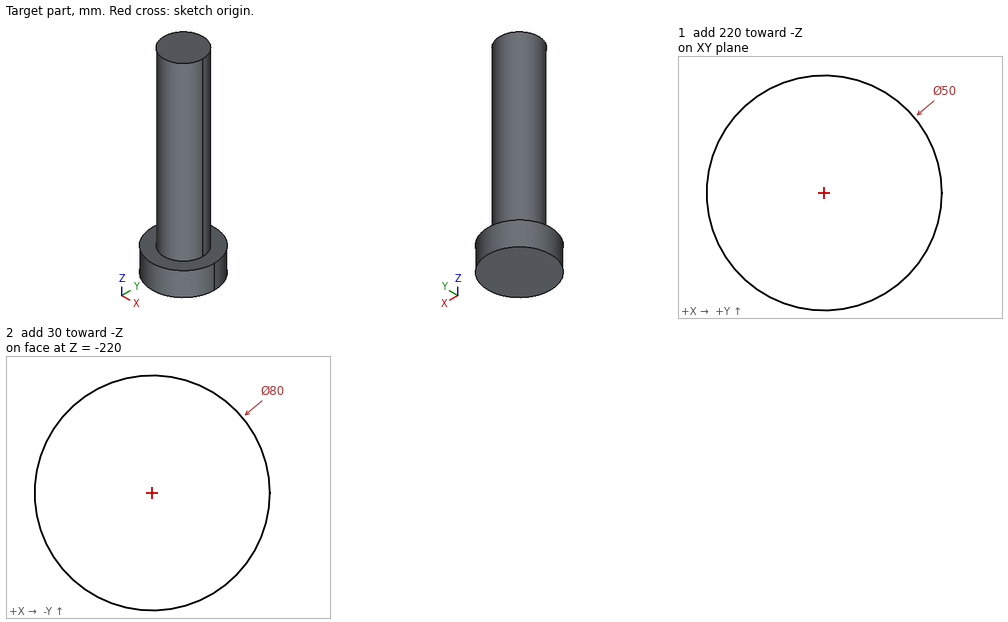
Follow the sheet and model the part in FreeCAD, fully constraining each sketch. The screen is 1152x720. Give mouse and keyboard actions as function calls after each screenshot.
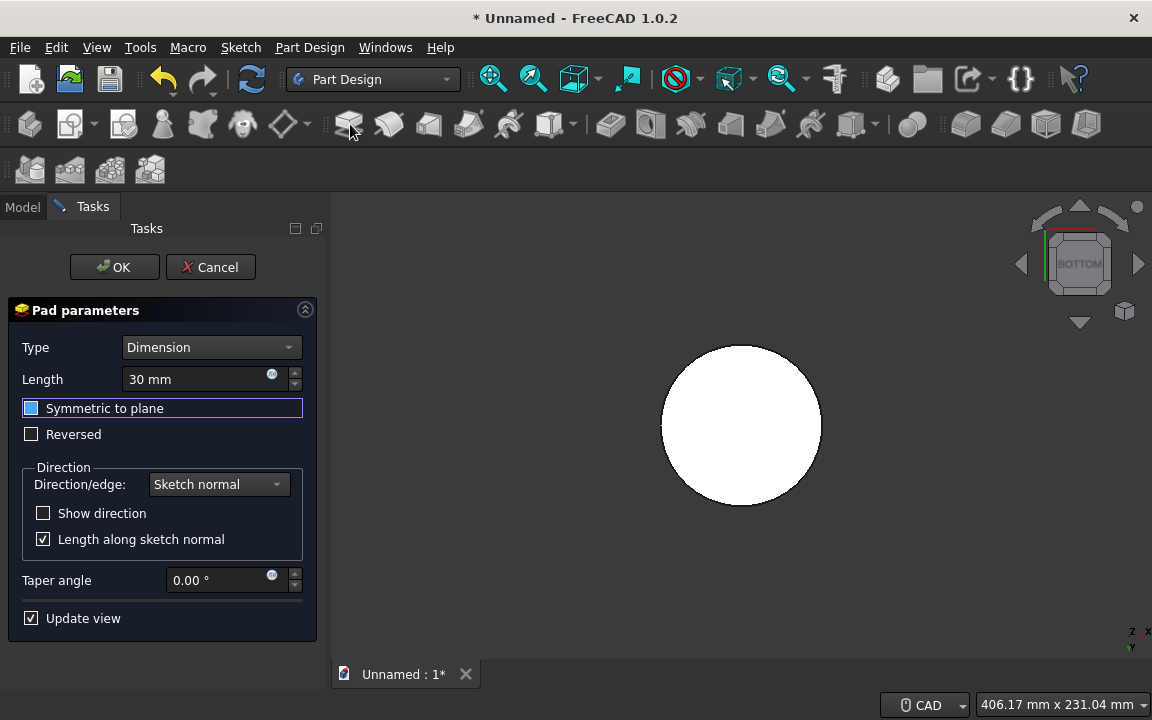
click(115, 267)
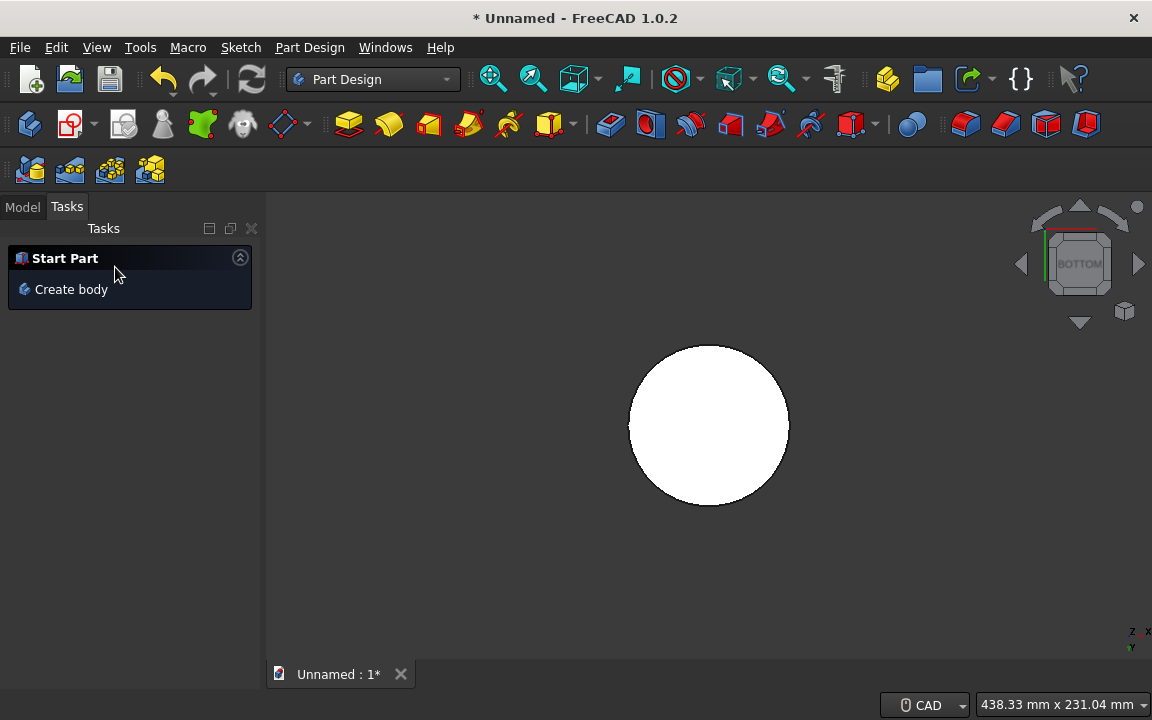
key(0)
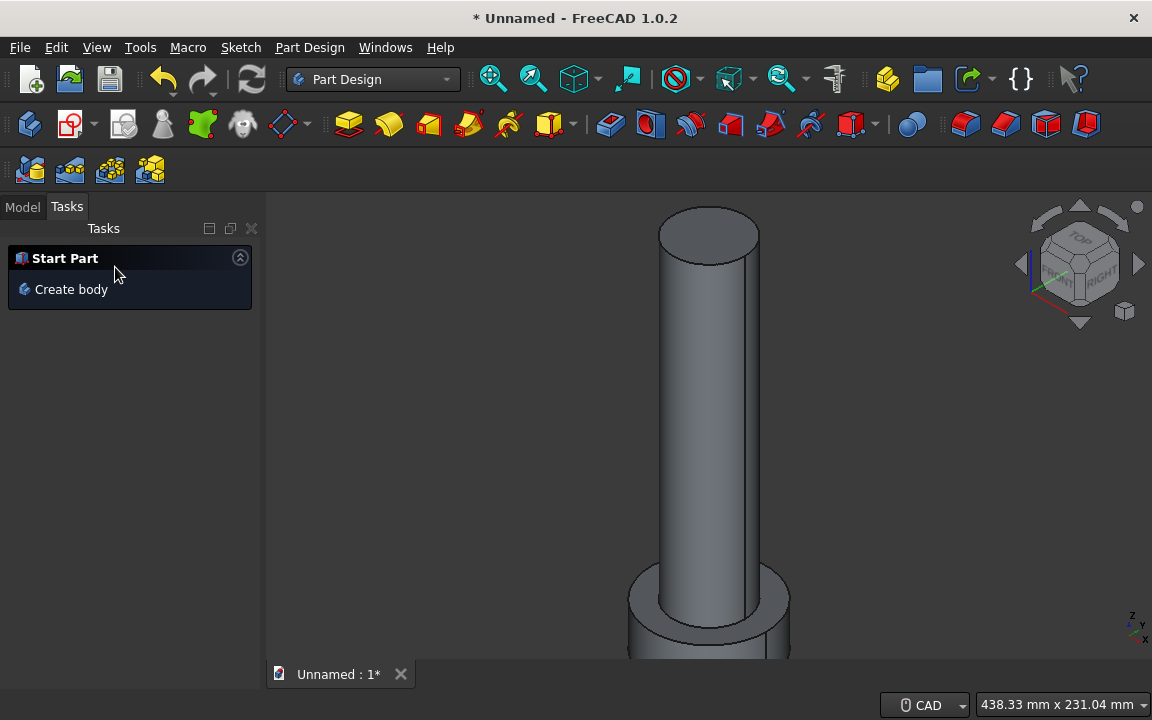
click(494, 80)